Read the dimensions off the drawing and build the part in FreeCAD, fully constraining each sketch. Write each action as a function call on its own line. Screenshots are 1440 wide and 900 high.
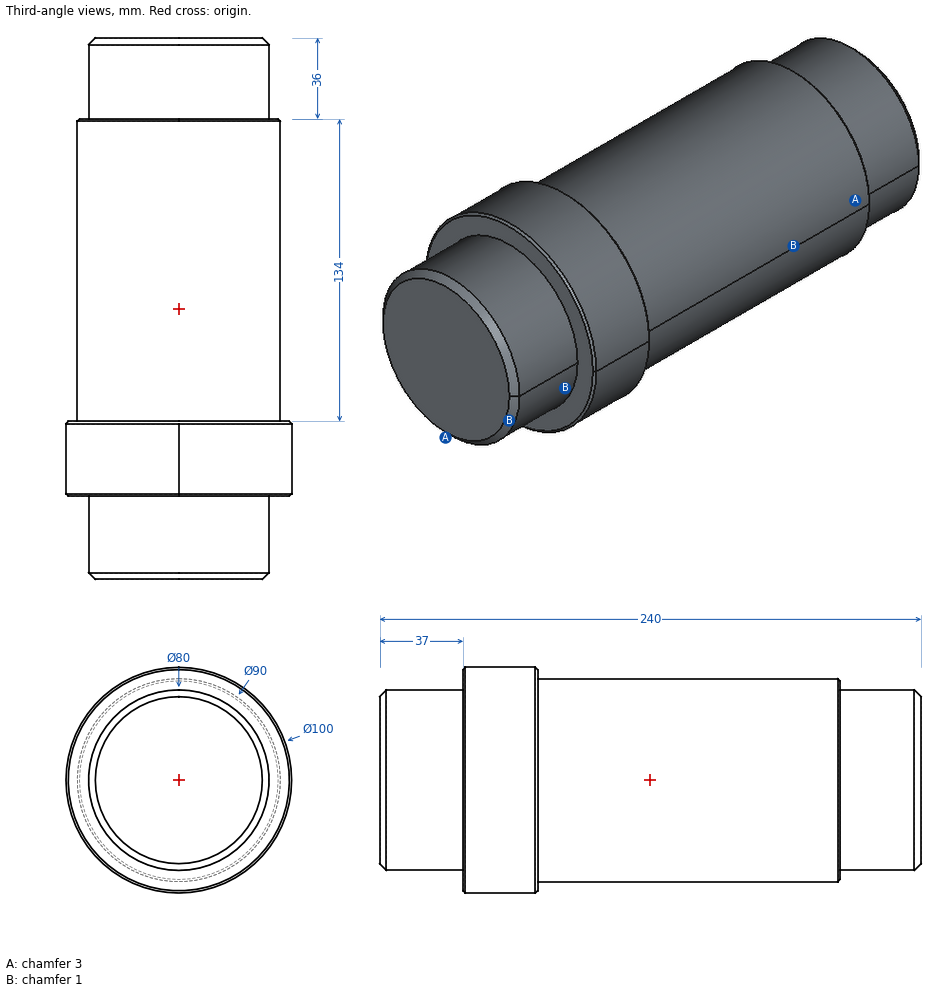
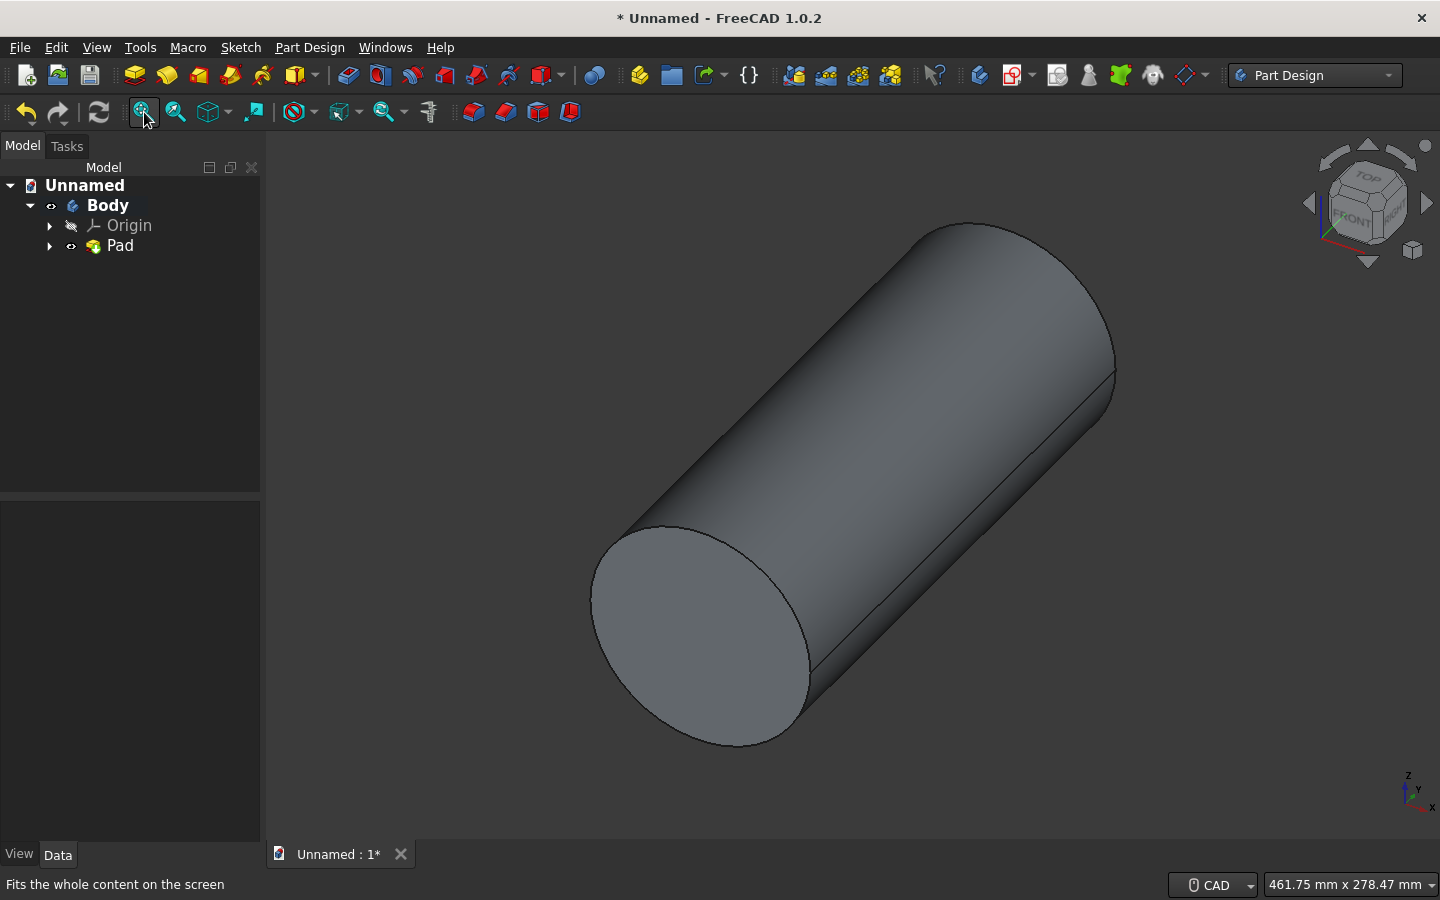
key(4)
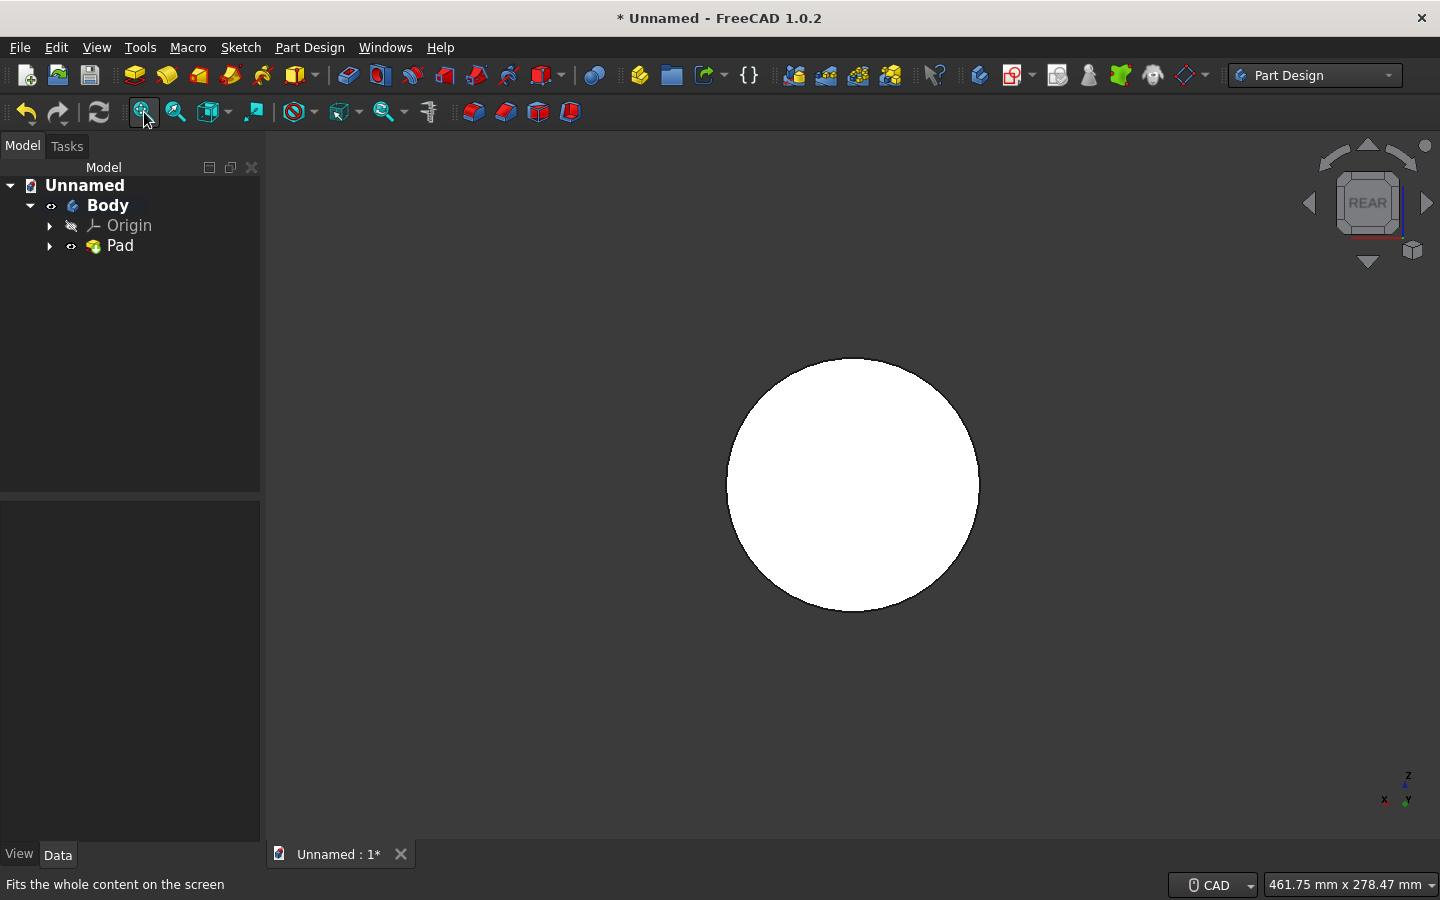
click(144, 112)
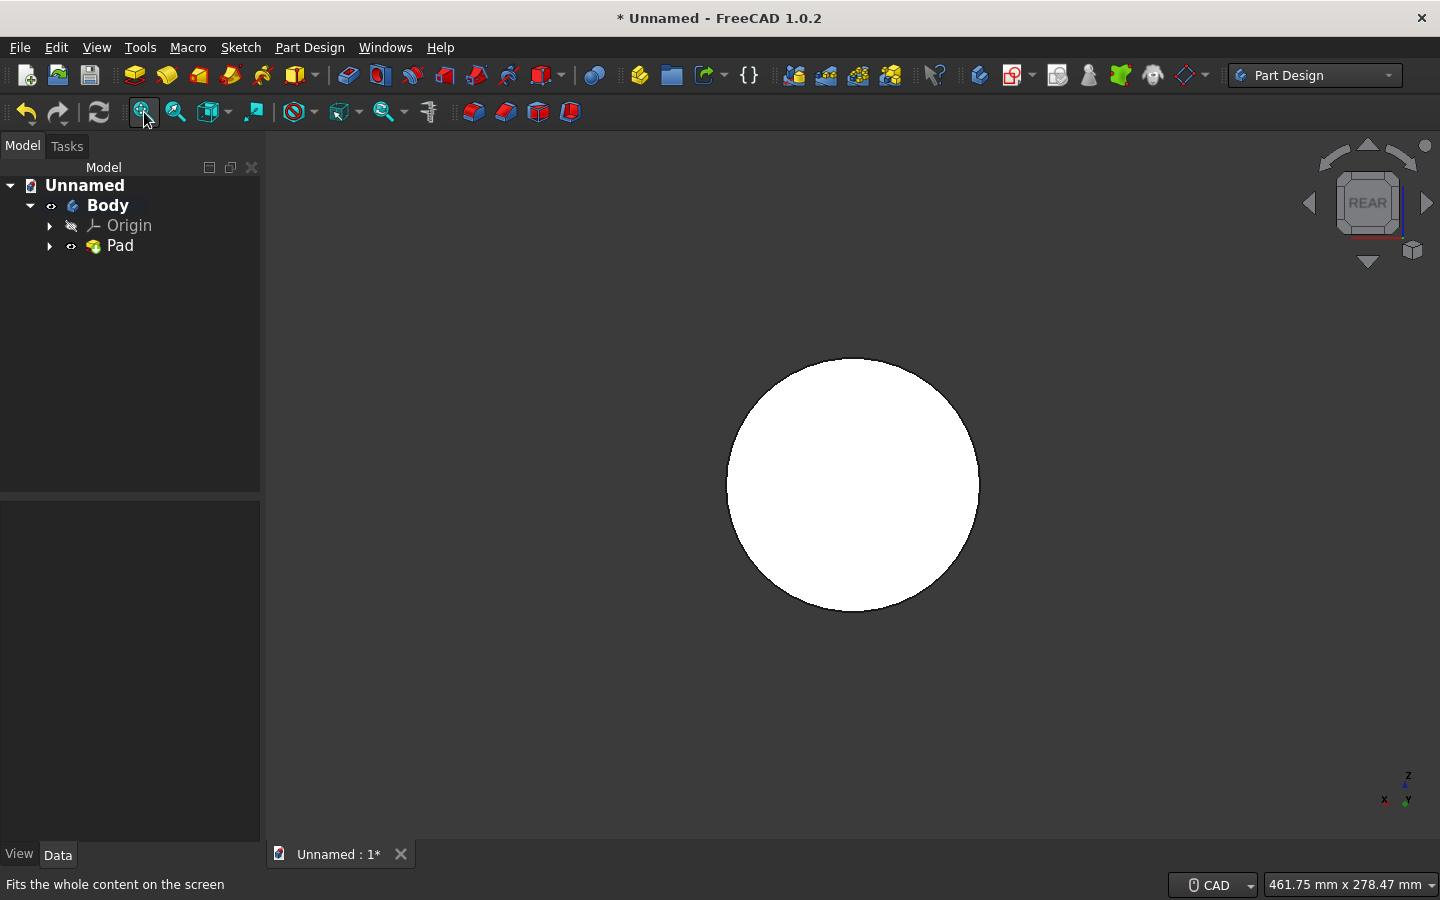
click(853, 484)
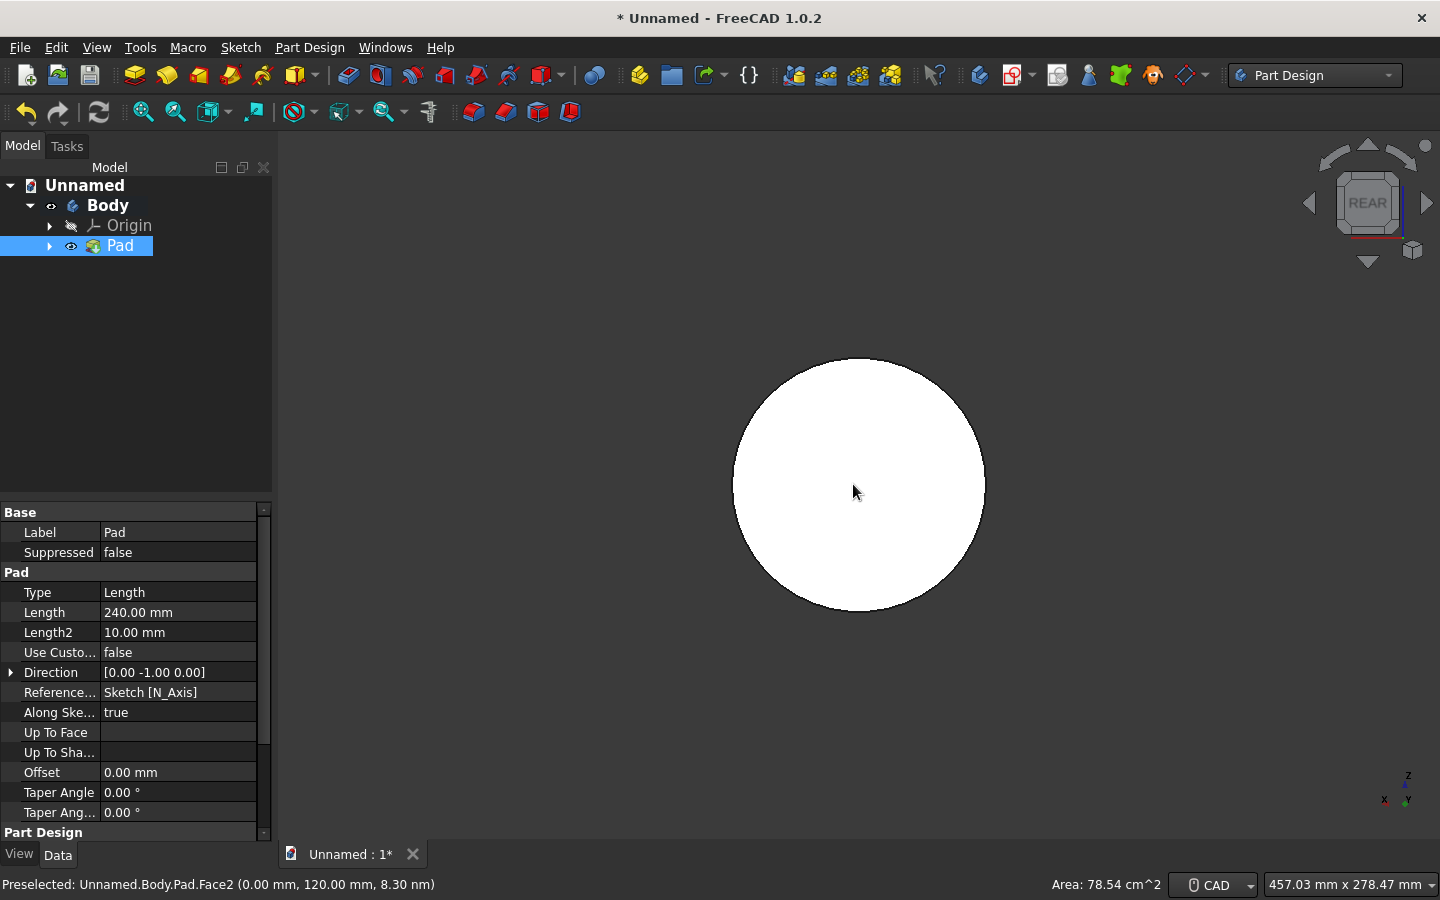
click(1012, 76)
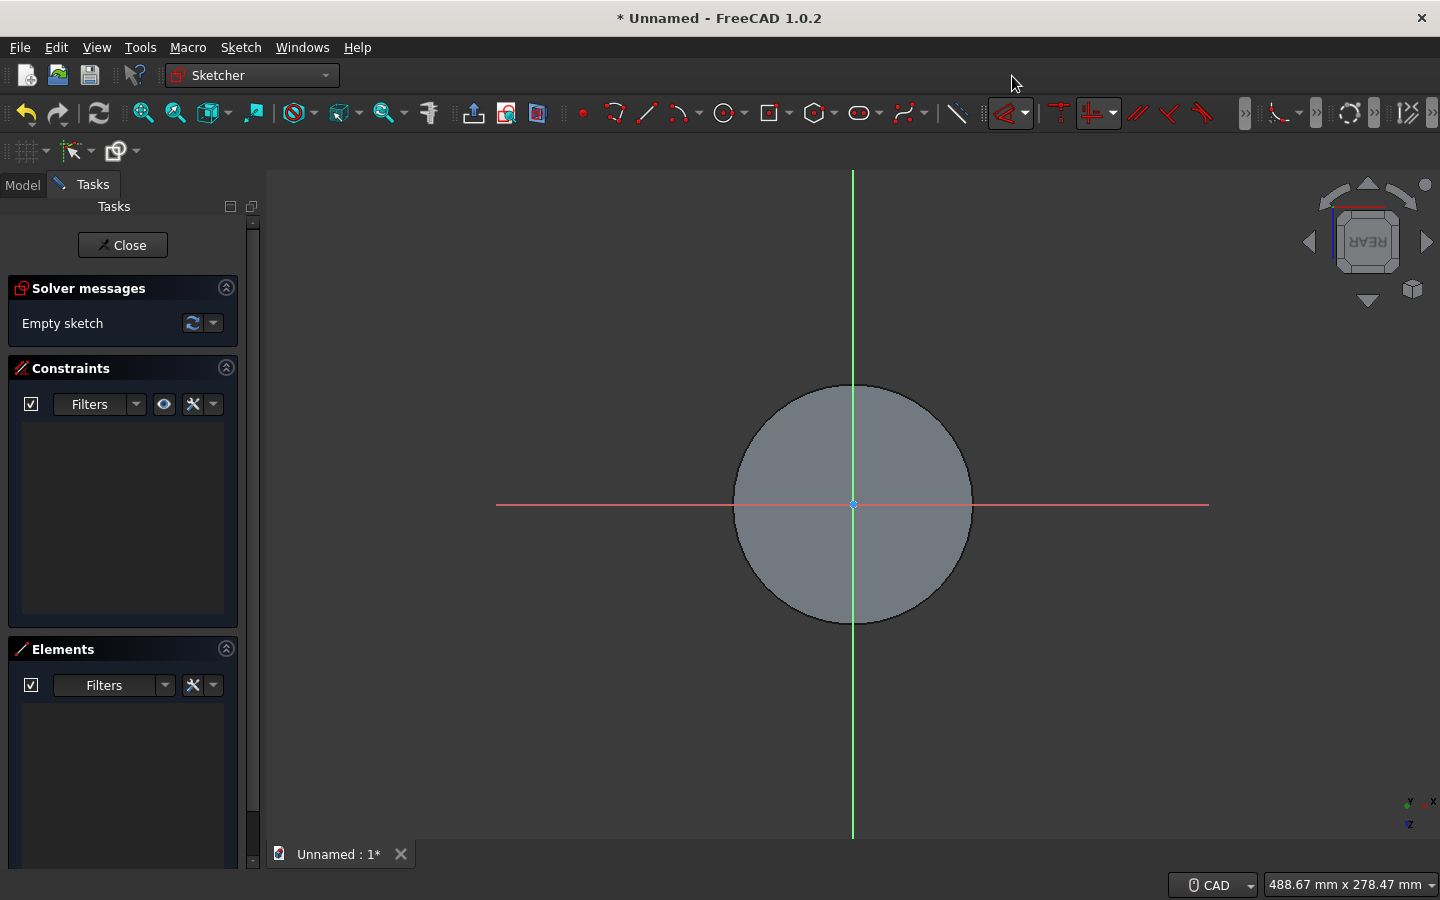
scroll(936, 504, up, 3)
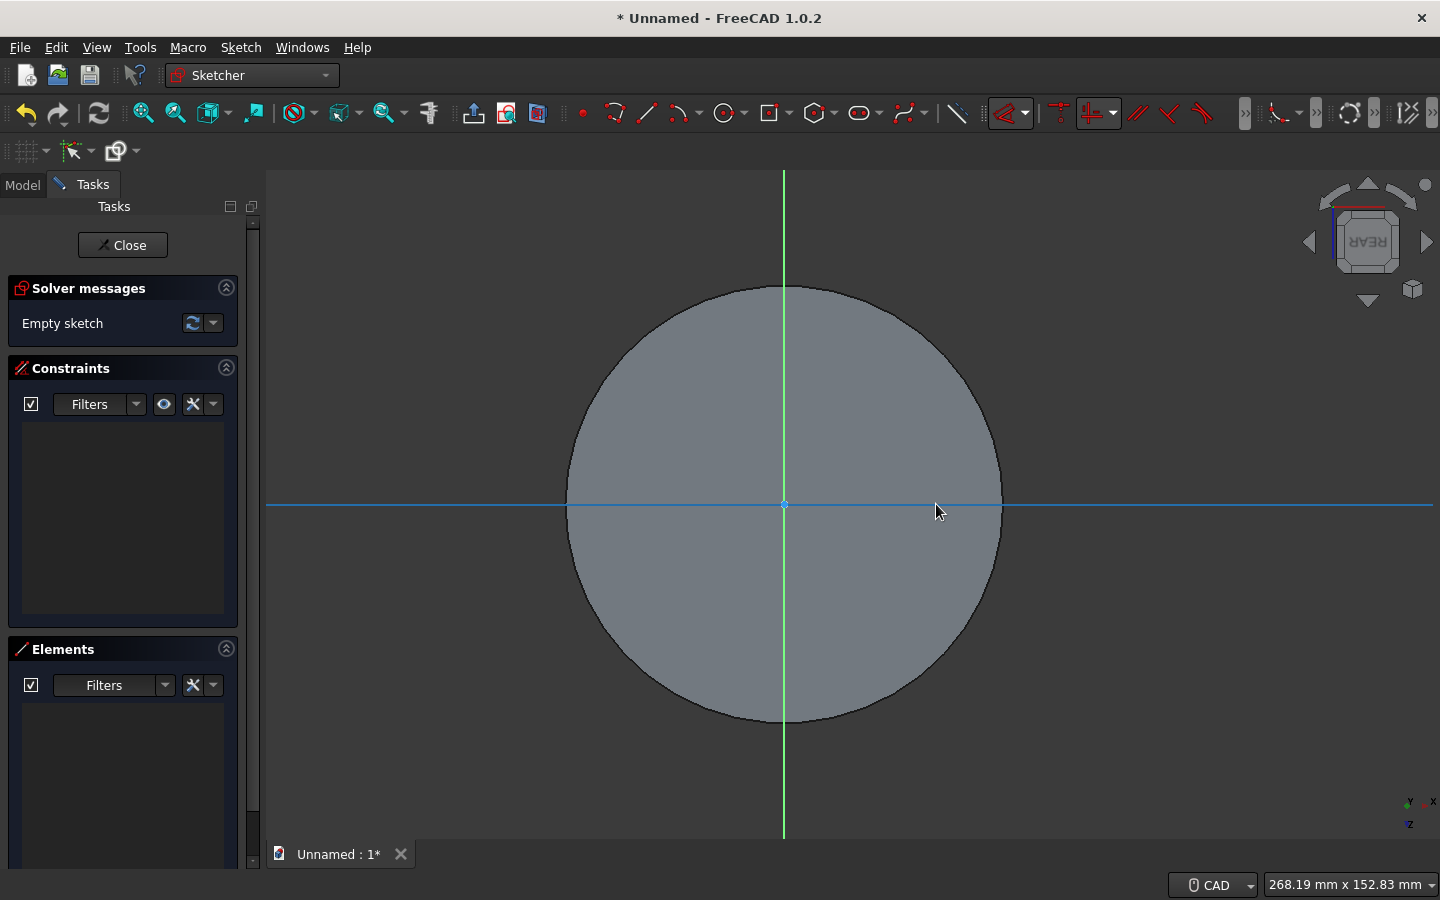
key(g)
key(c)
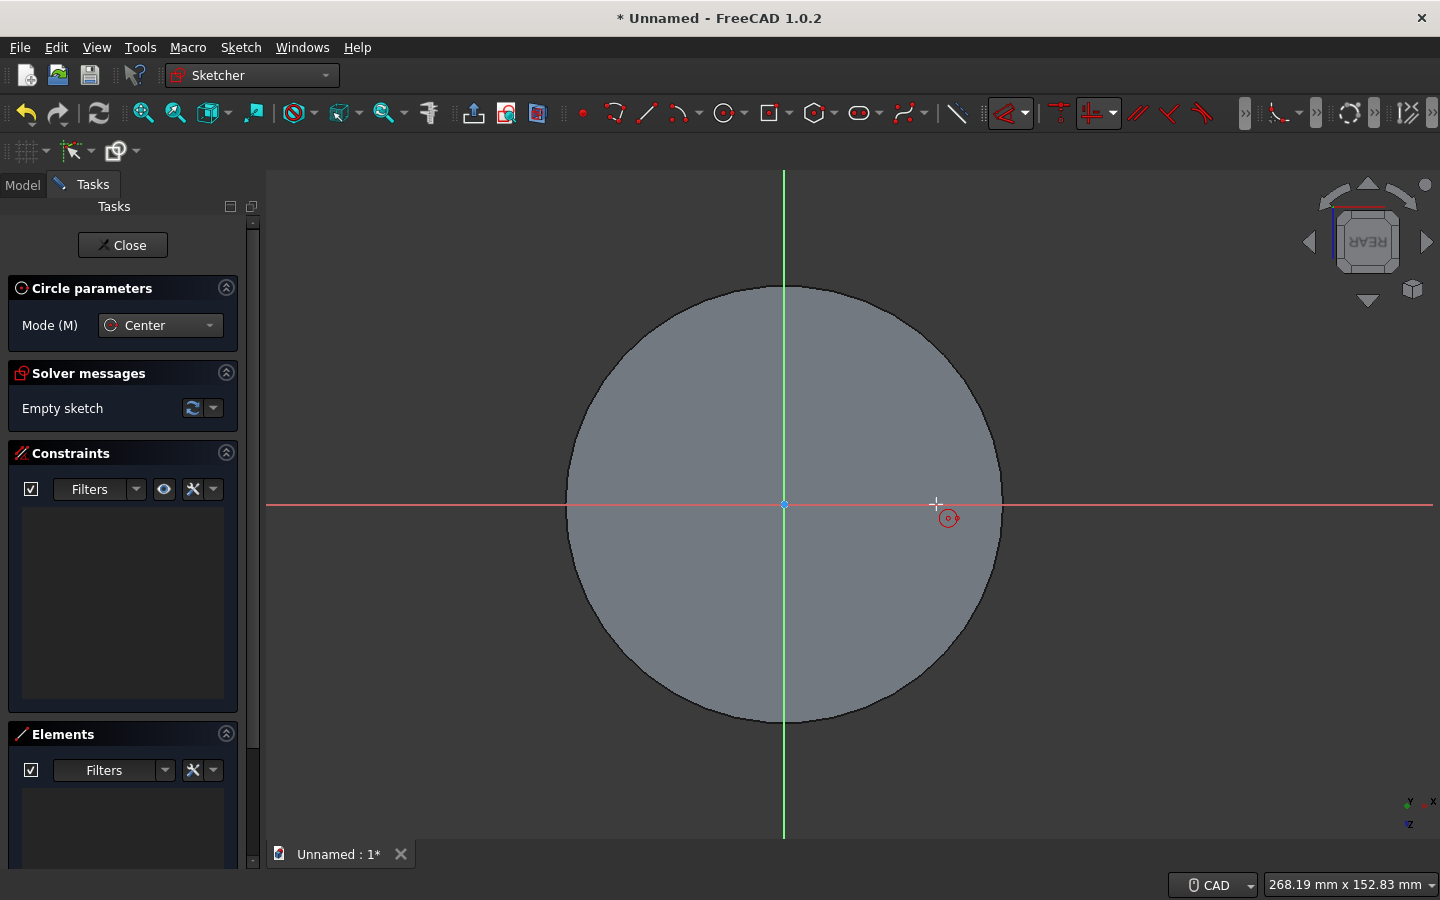
click(784, 504)
click(939, 350)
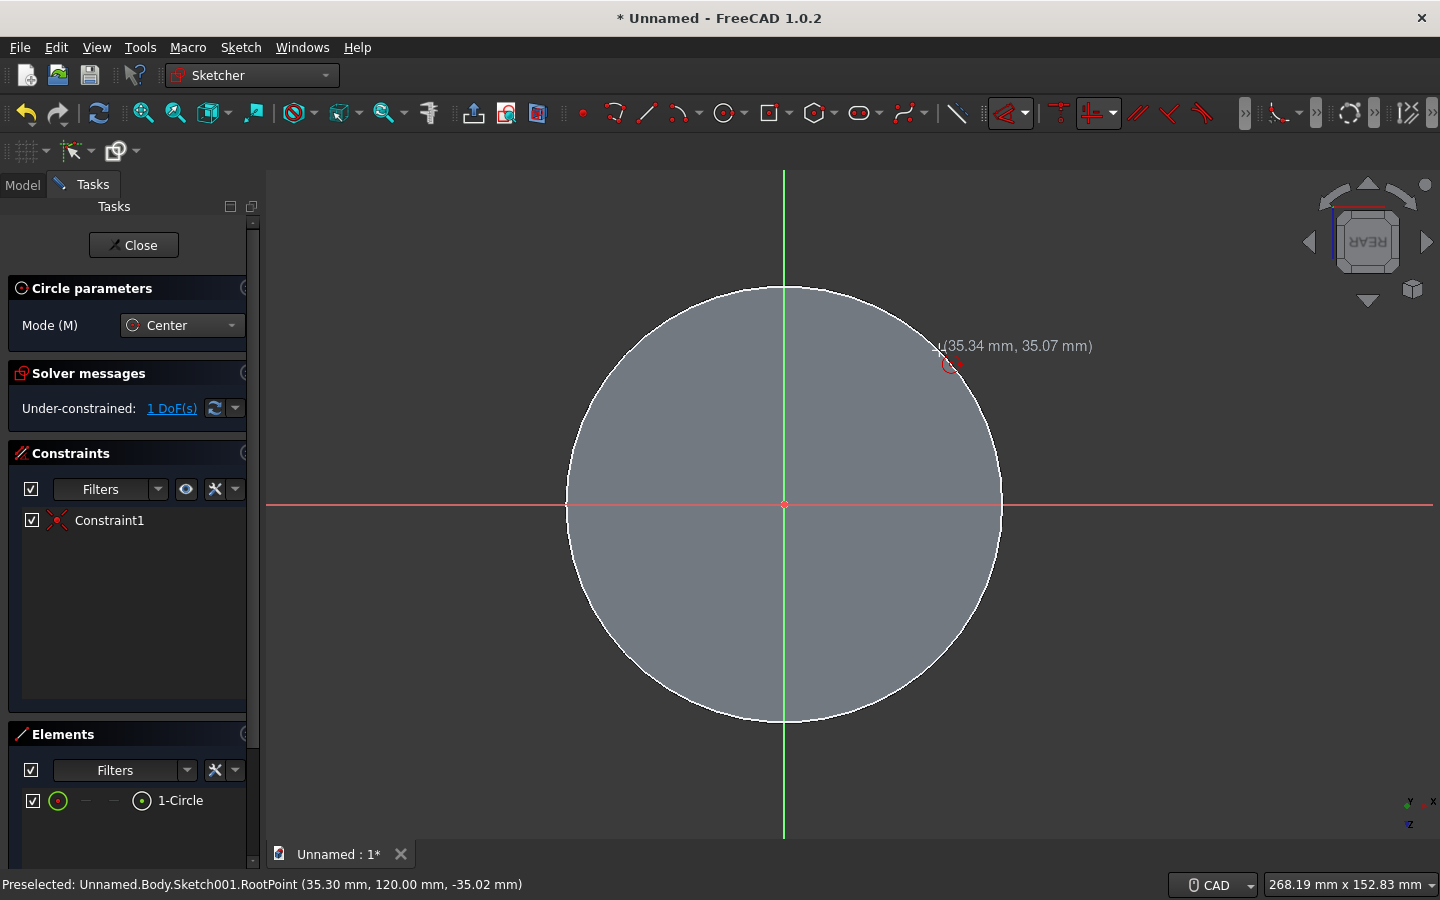
click(784, 504)
click(908, 381)
key(Escape)